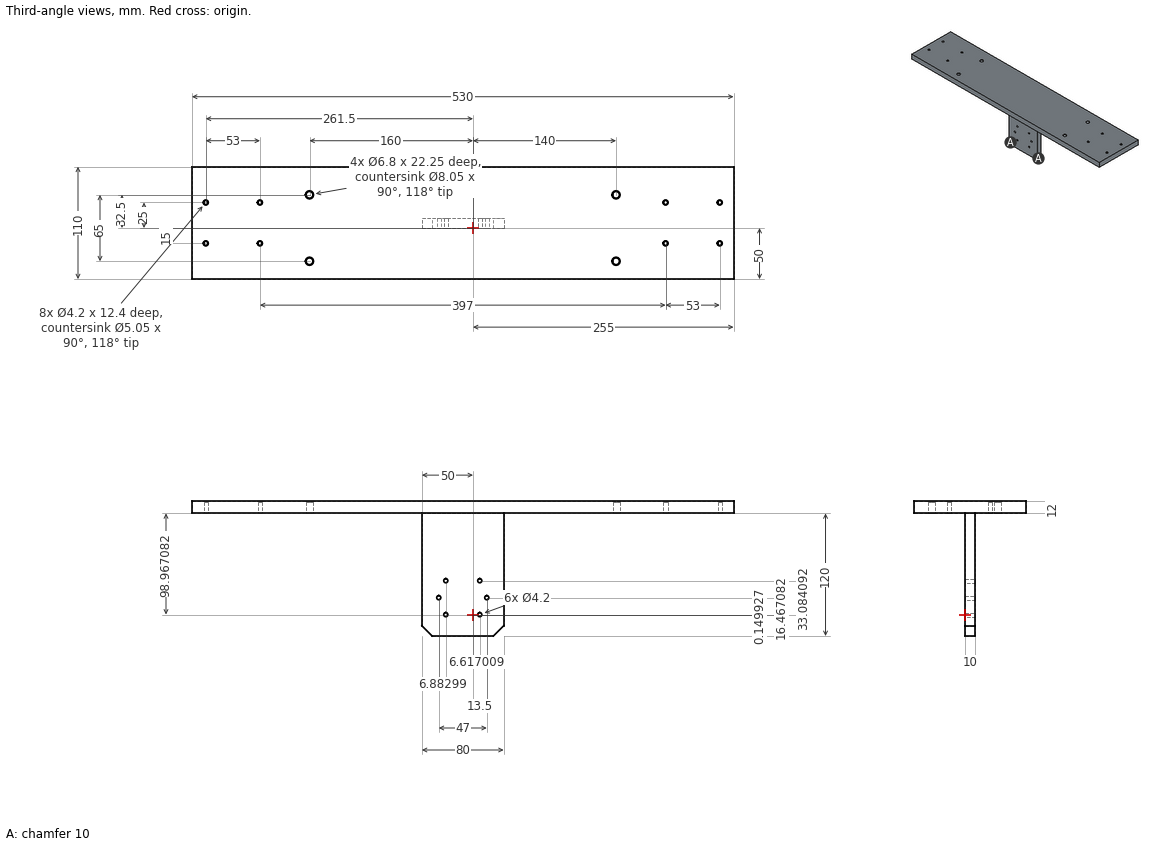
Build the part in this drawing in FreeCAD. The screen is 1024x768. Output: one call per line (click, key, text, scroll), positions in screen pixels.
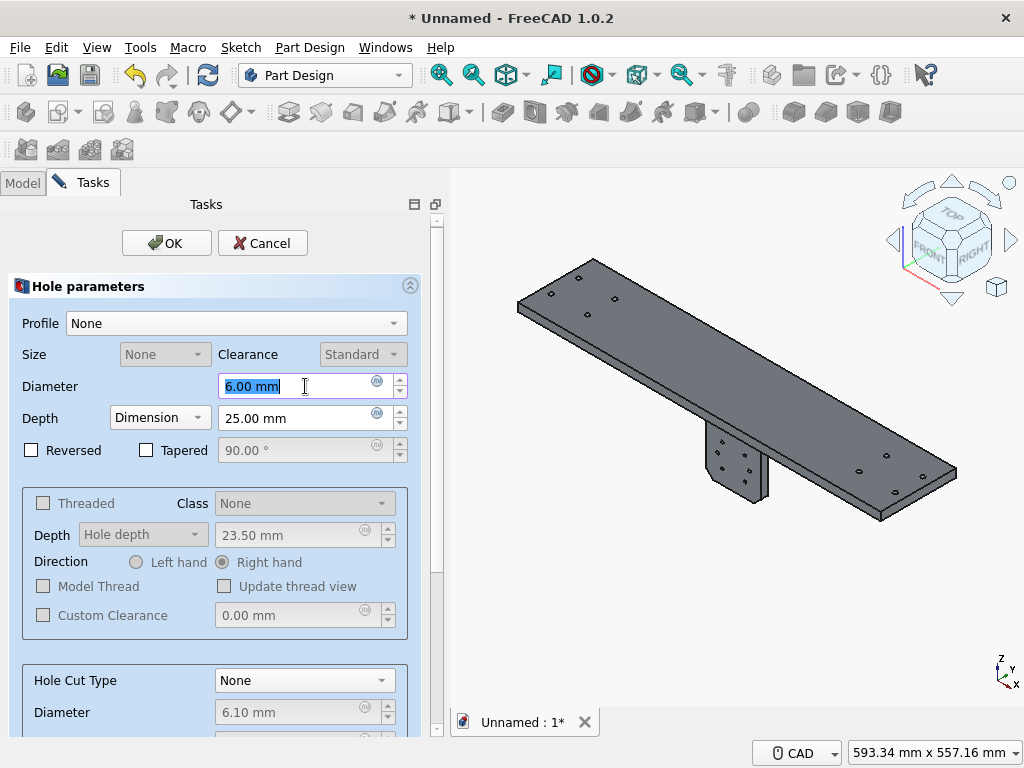
text(4.2)
key(Tab)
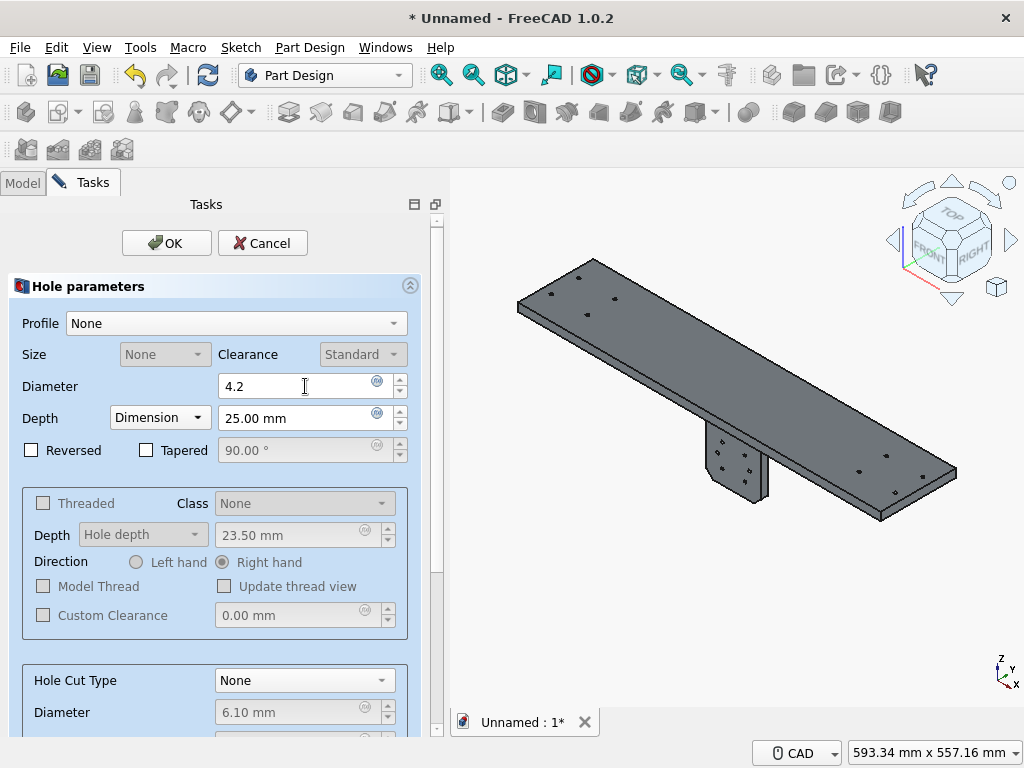
triple_click(305, 418)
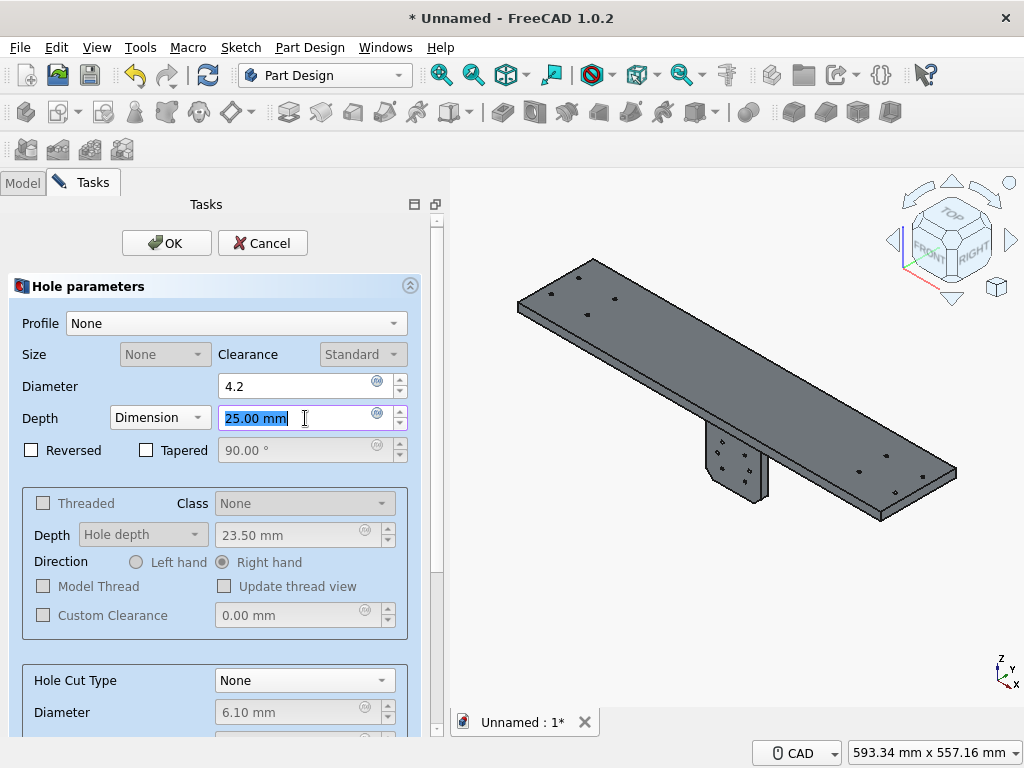
text(12.4)
key(Tab)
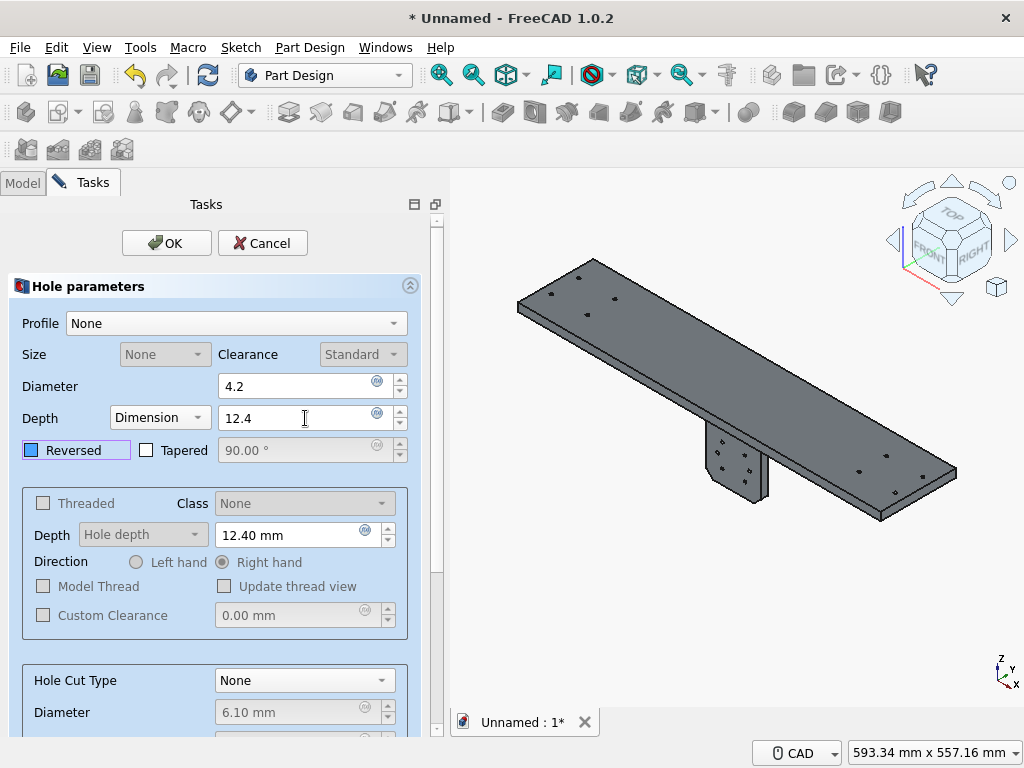
click(306, 680)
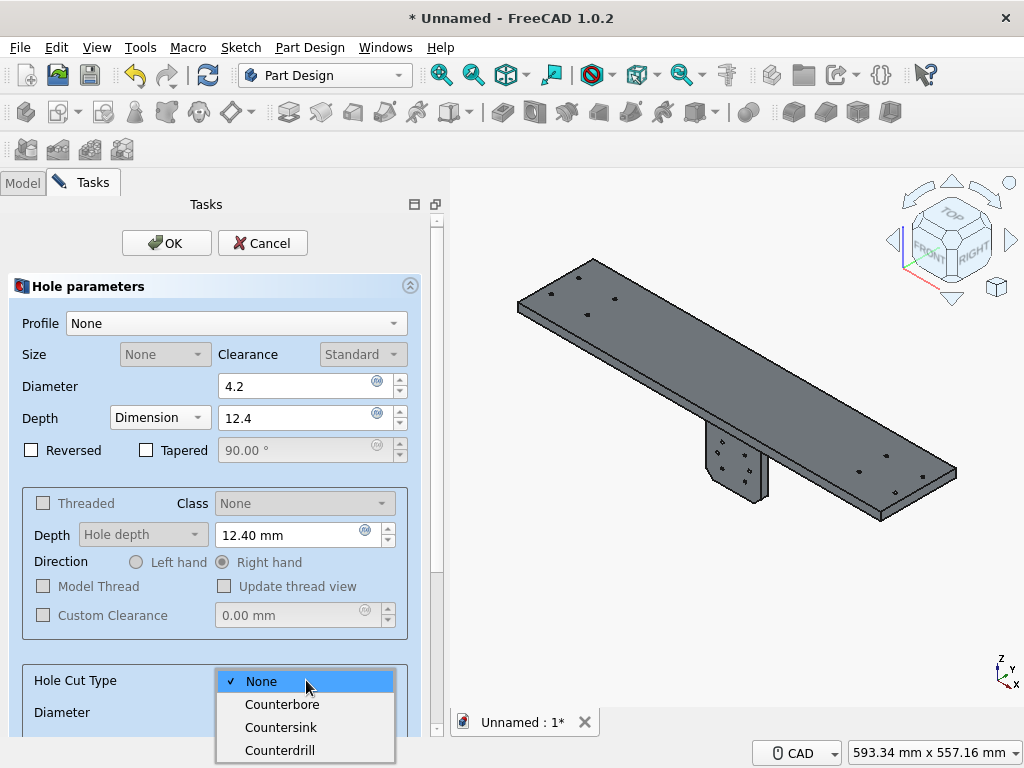
click(304, 728)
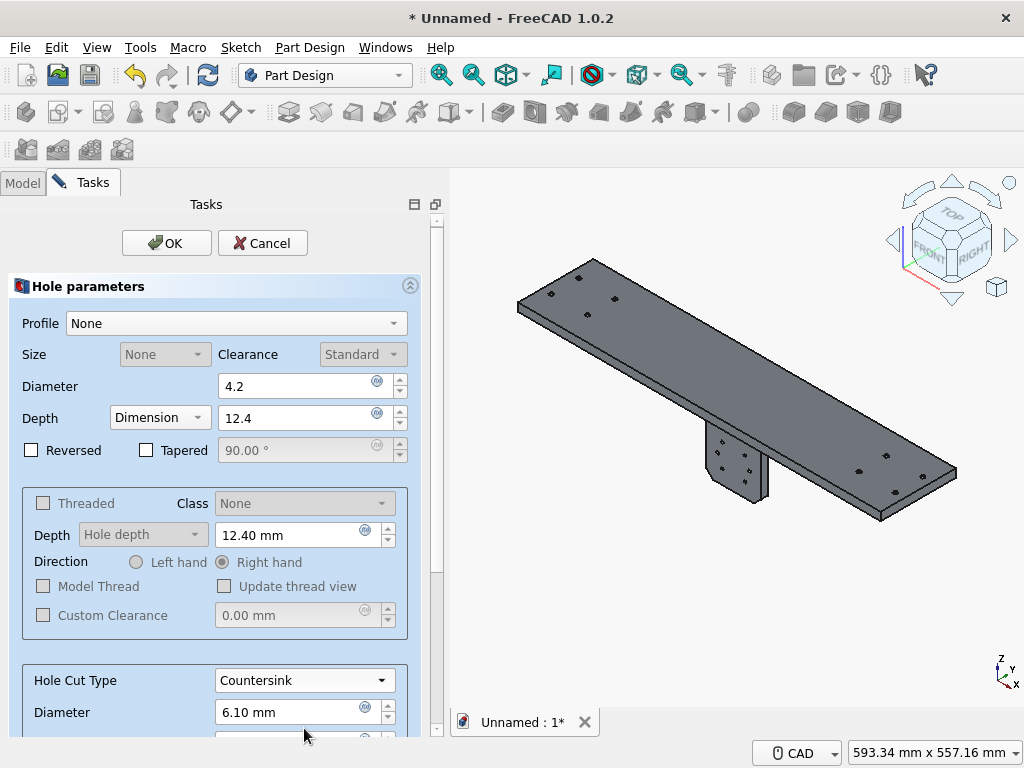
triple_click(298, 712)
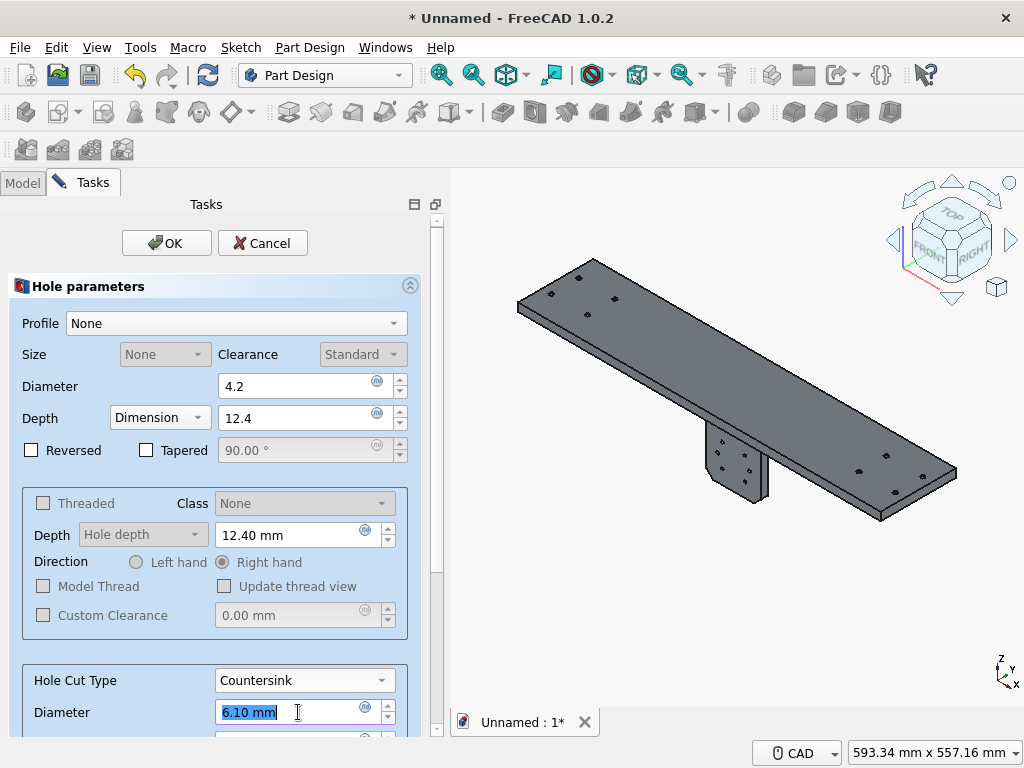
text(5.05)
key(Tab)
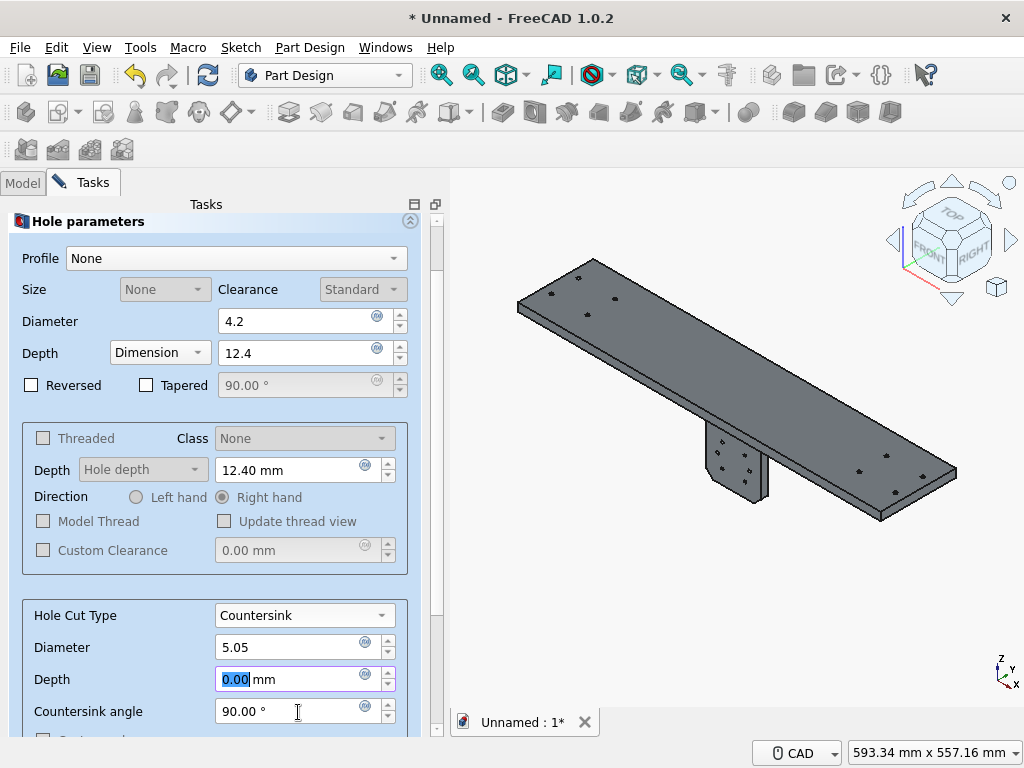
scroll(437, 475, up, 2)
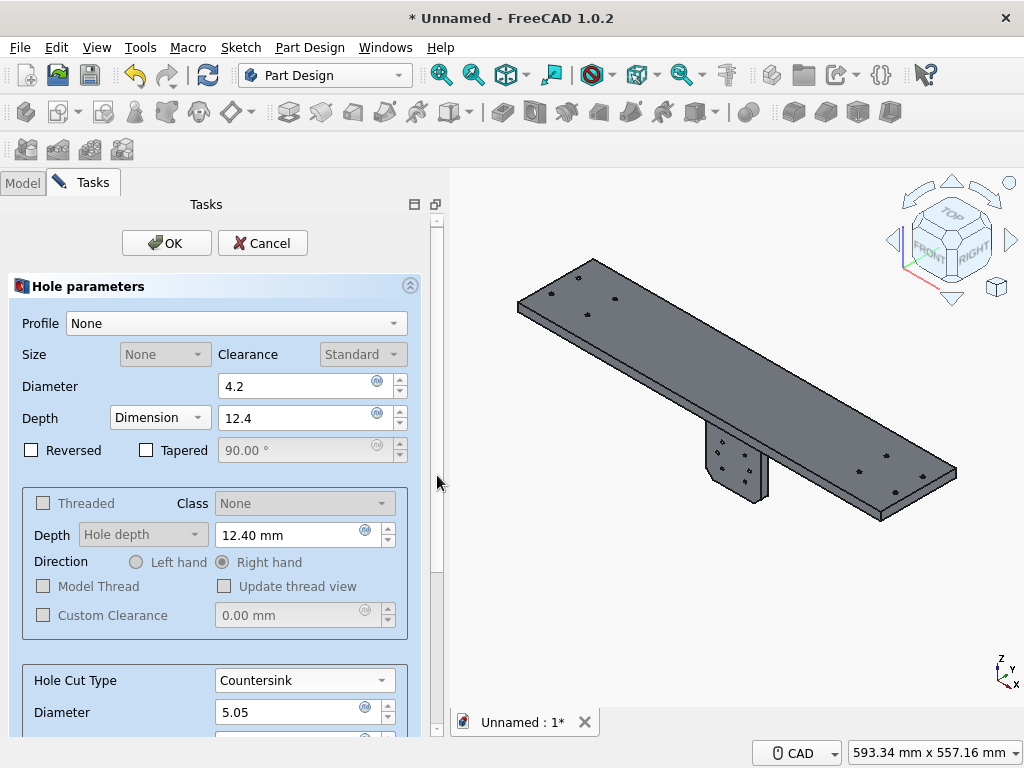
click(167, 243)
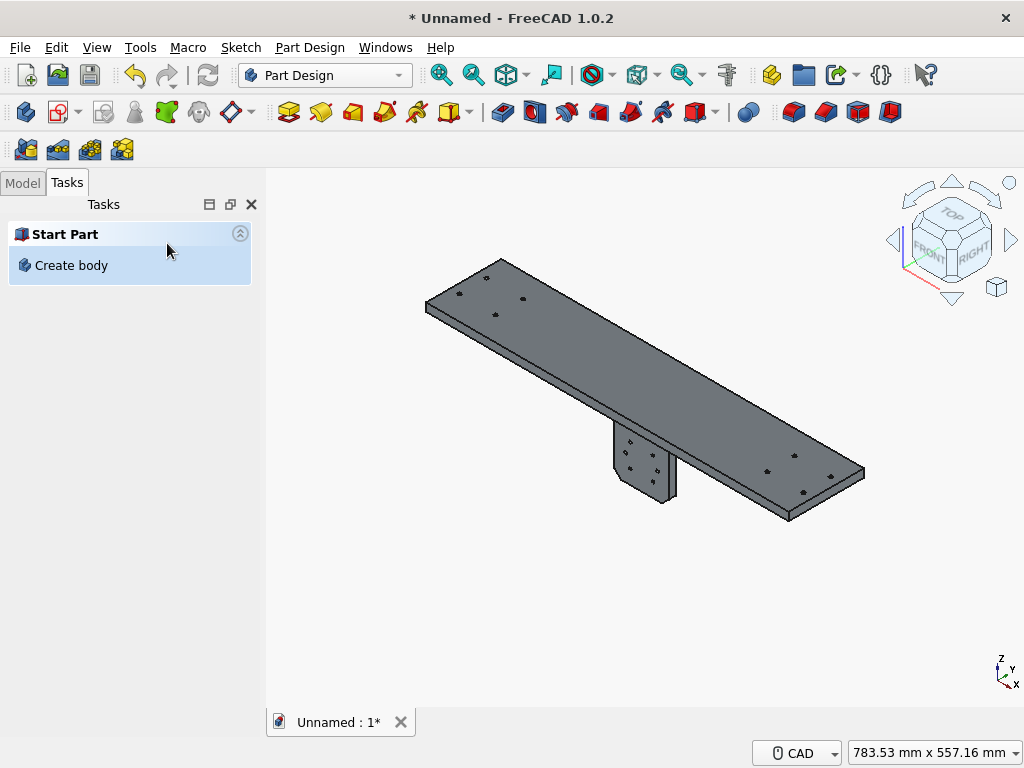
click(697, 414)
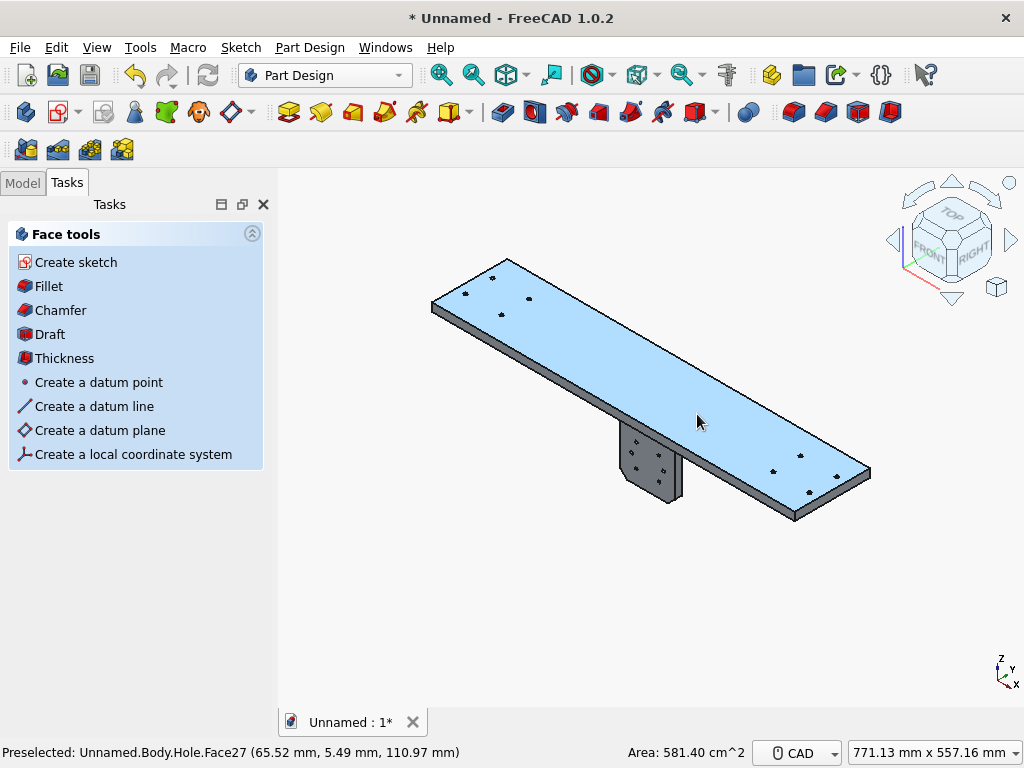
click(58, 112)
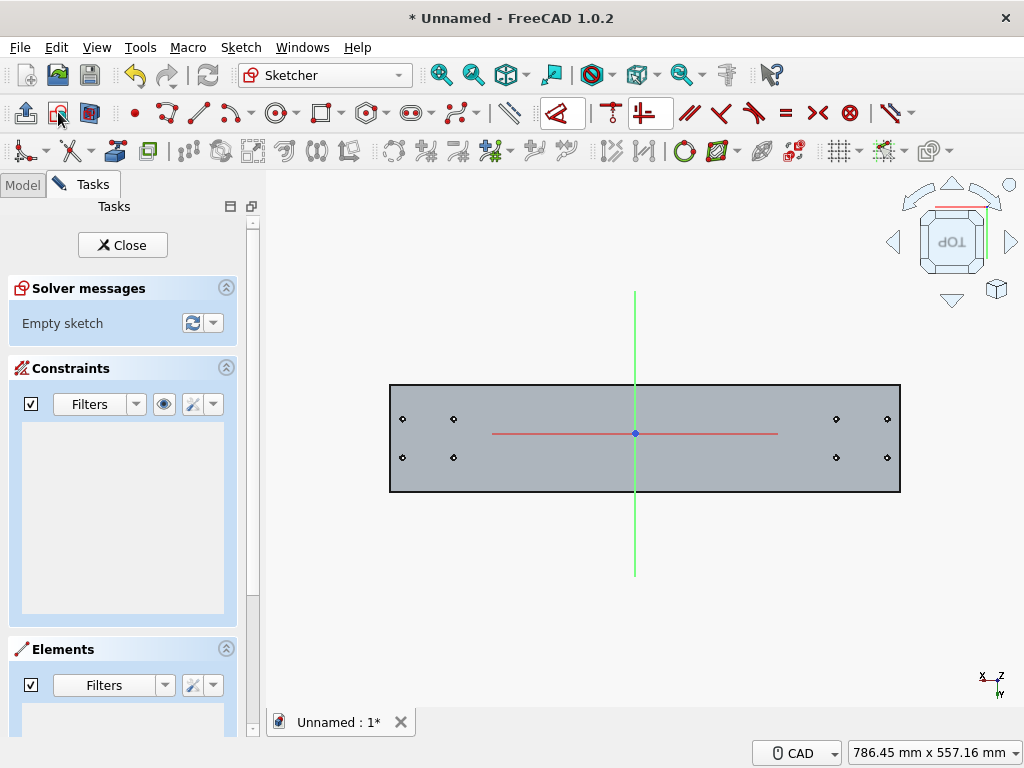
key(g)
key(c)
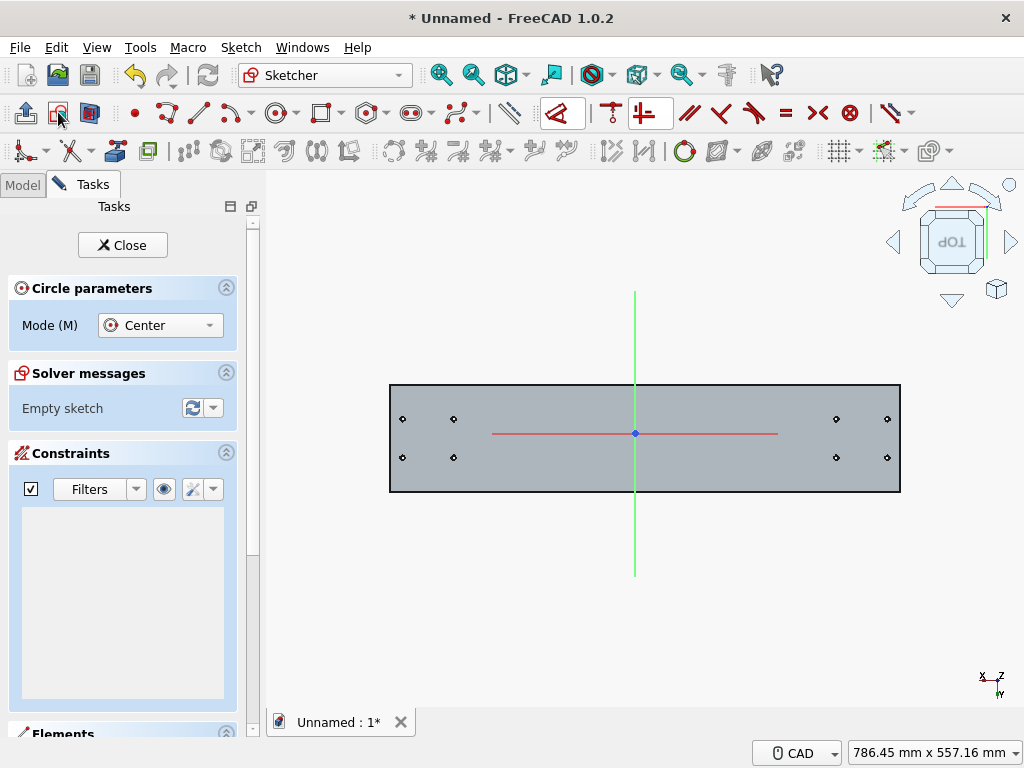
scroll(790, 465, up, 10)